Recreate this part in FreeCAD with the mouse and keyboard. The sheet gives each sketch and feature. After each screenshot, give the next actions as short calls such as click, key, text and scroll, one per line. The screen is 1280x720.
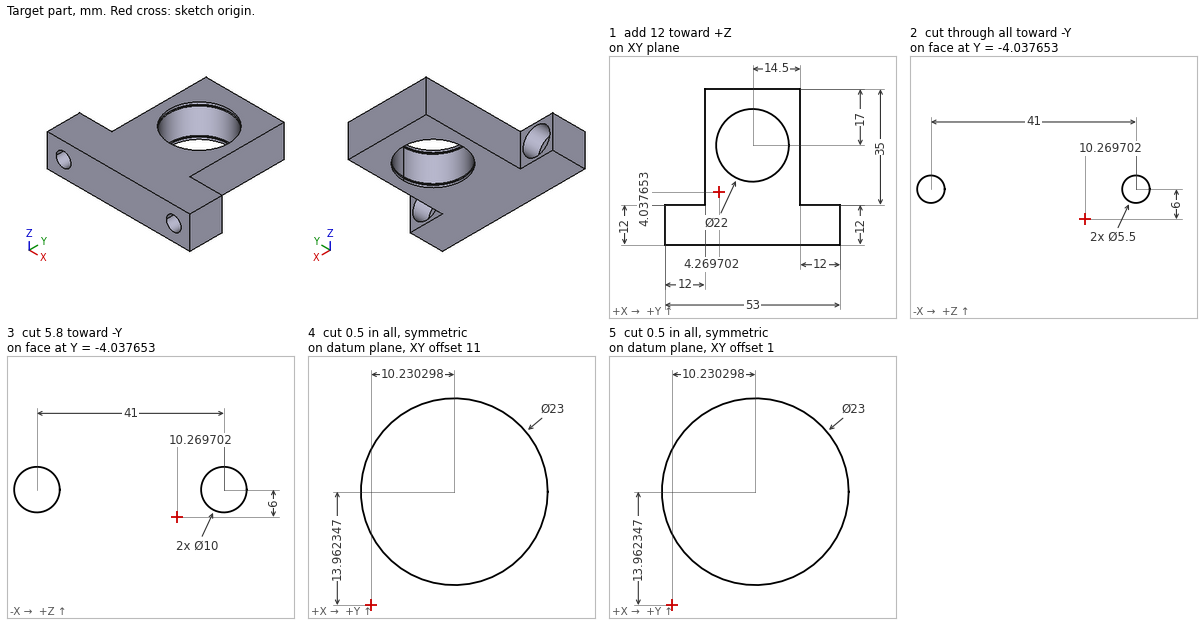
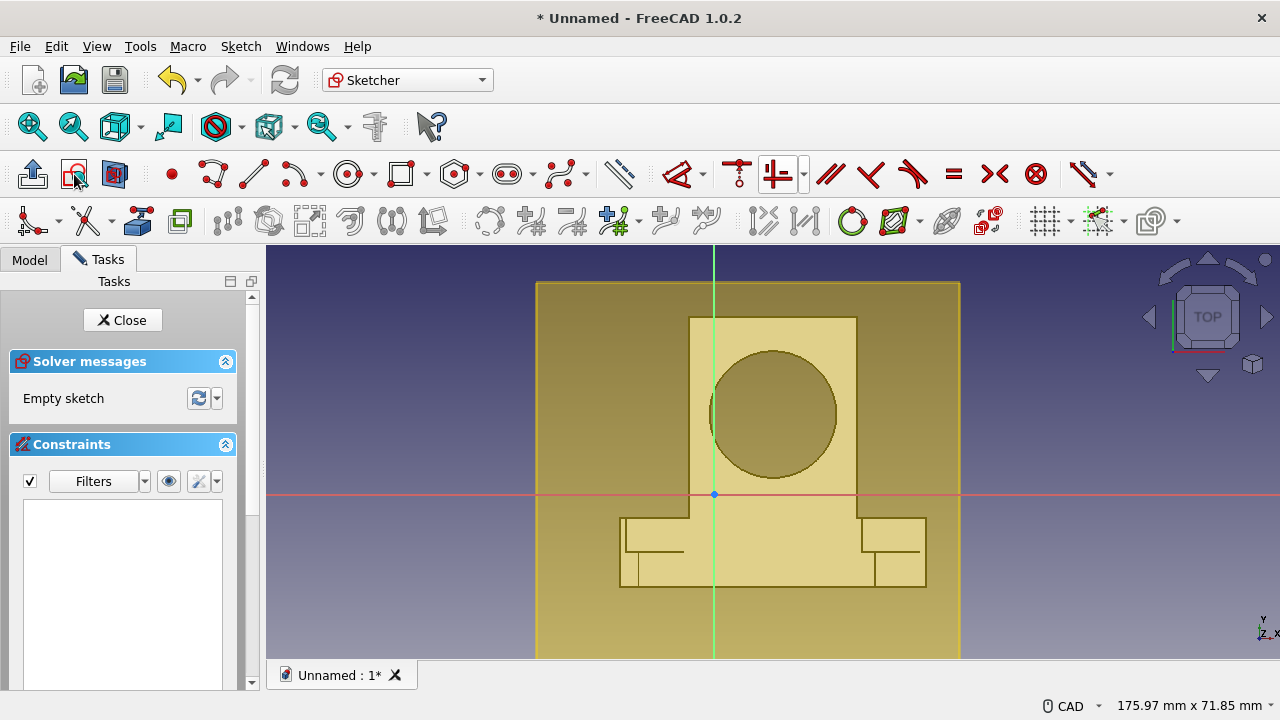
scroll(856, 385, up, 3)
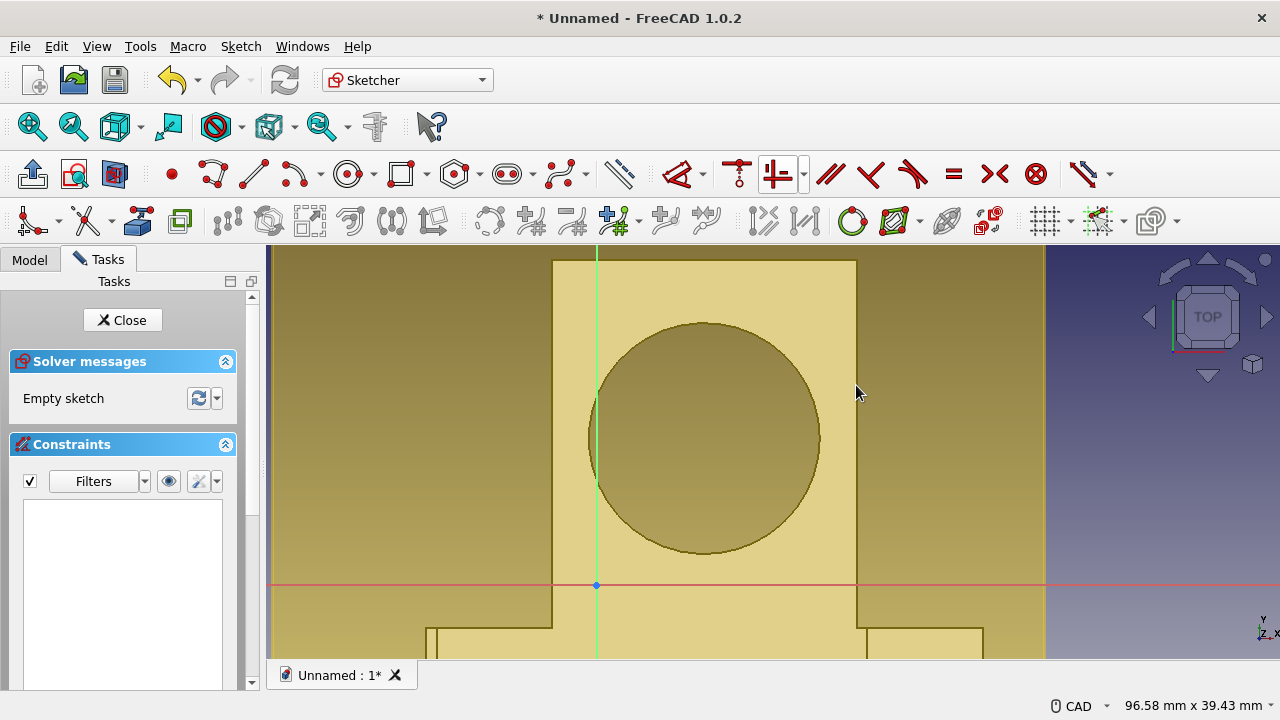
click(348, 174)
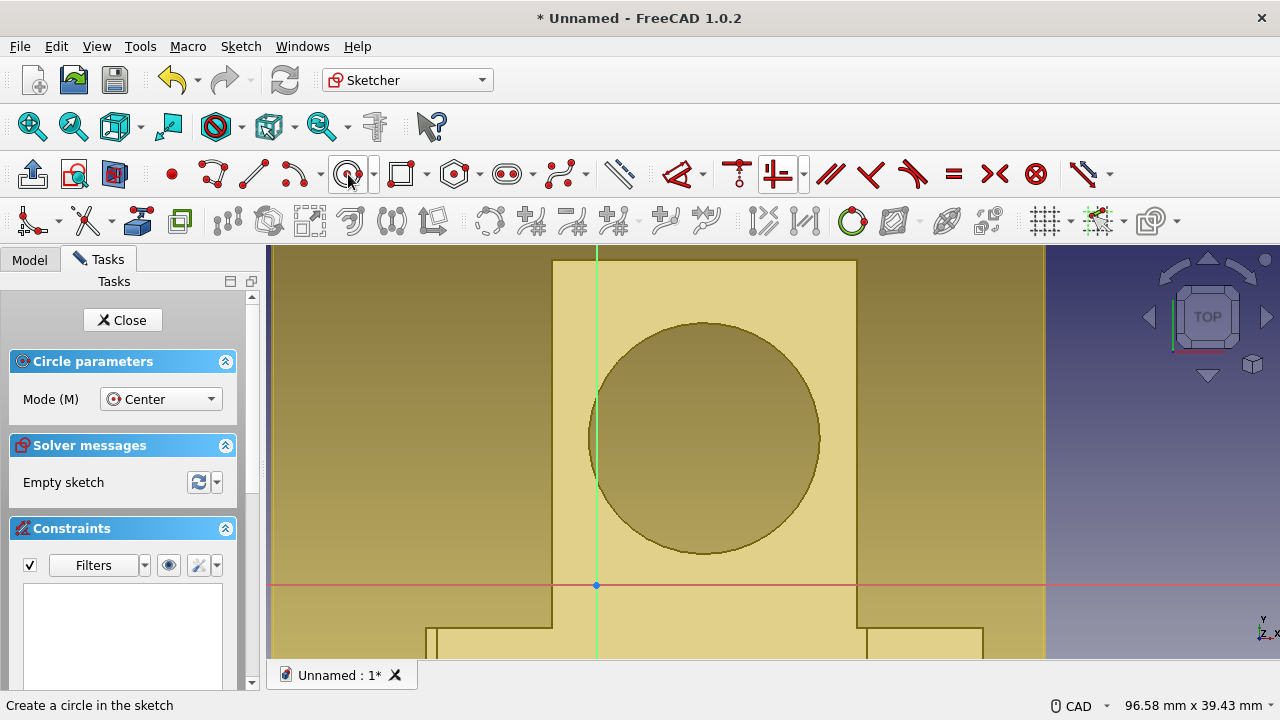
click(704, 439)
click(790, 353)
key(Escape)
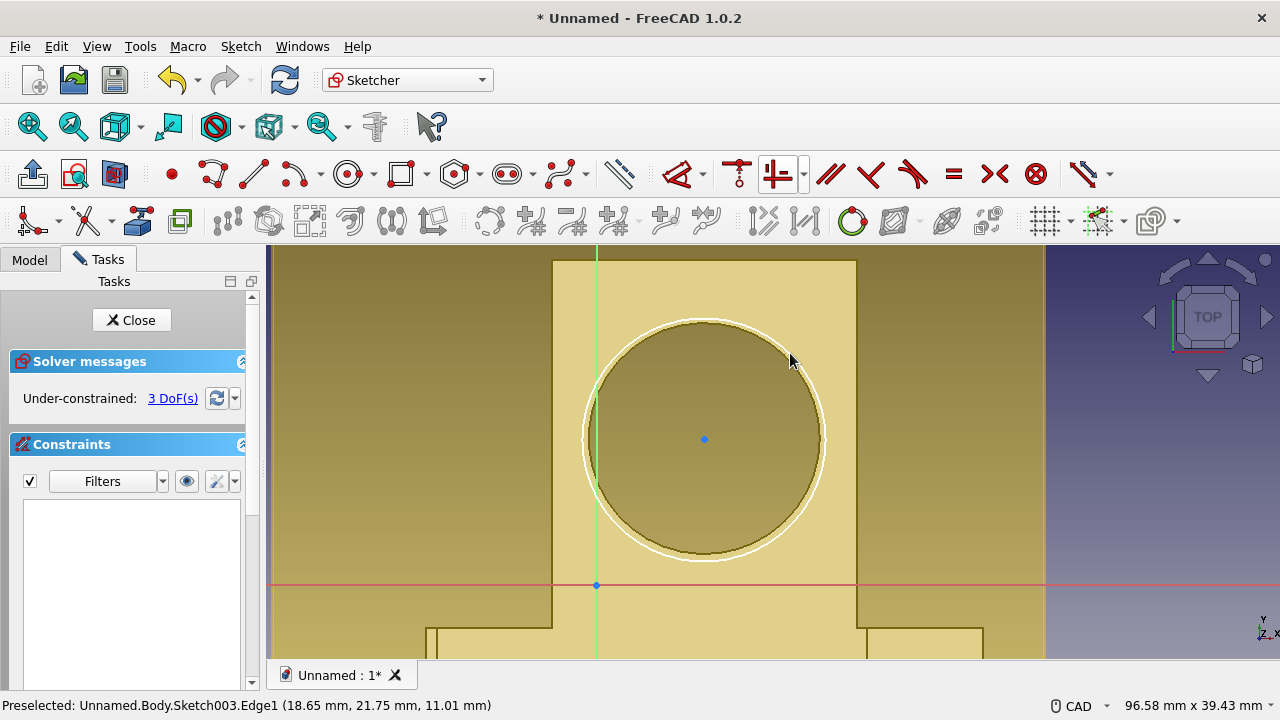
key(d)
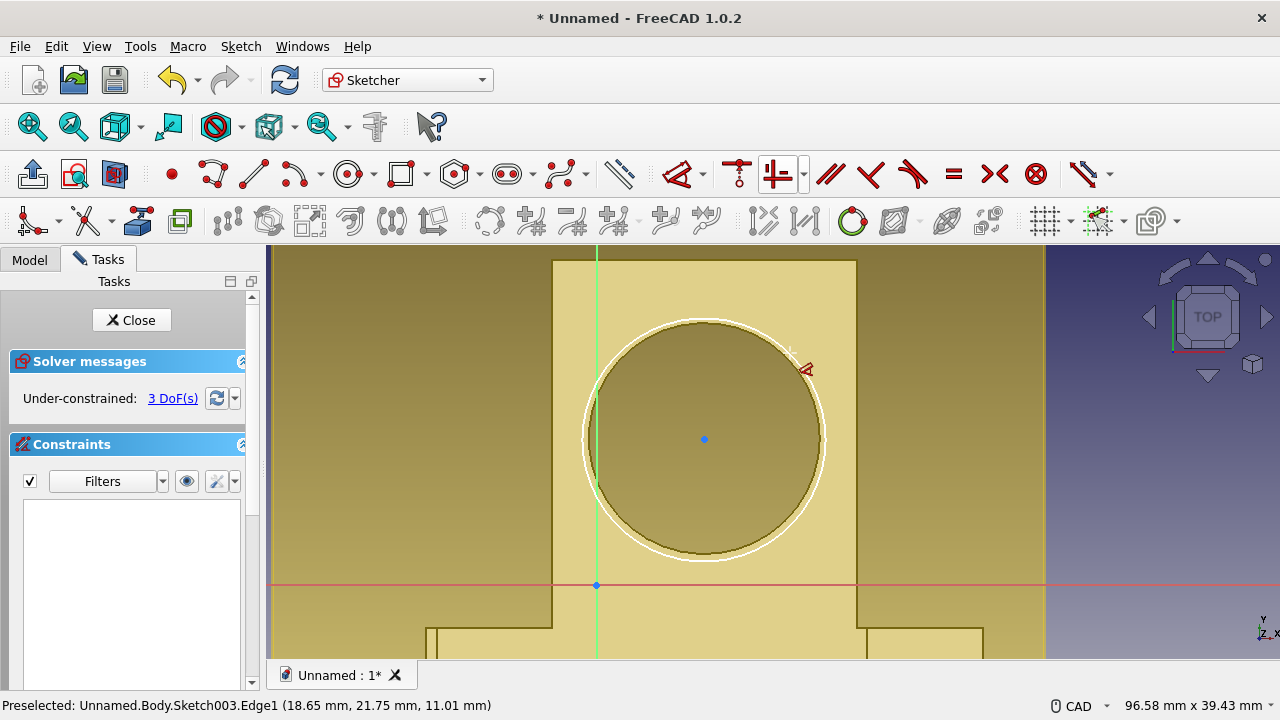
click(790, 354)
click(813, 331)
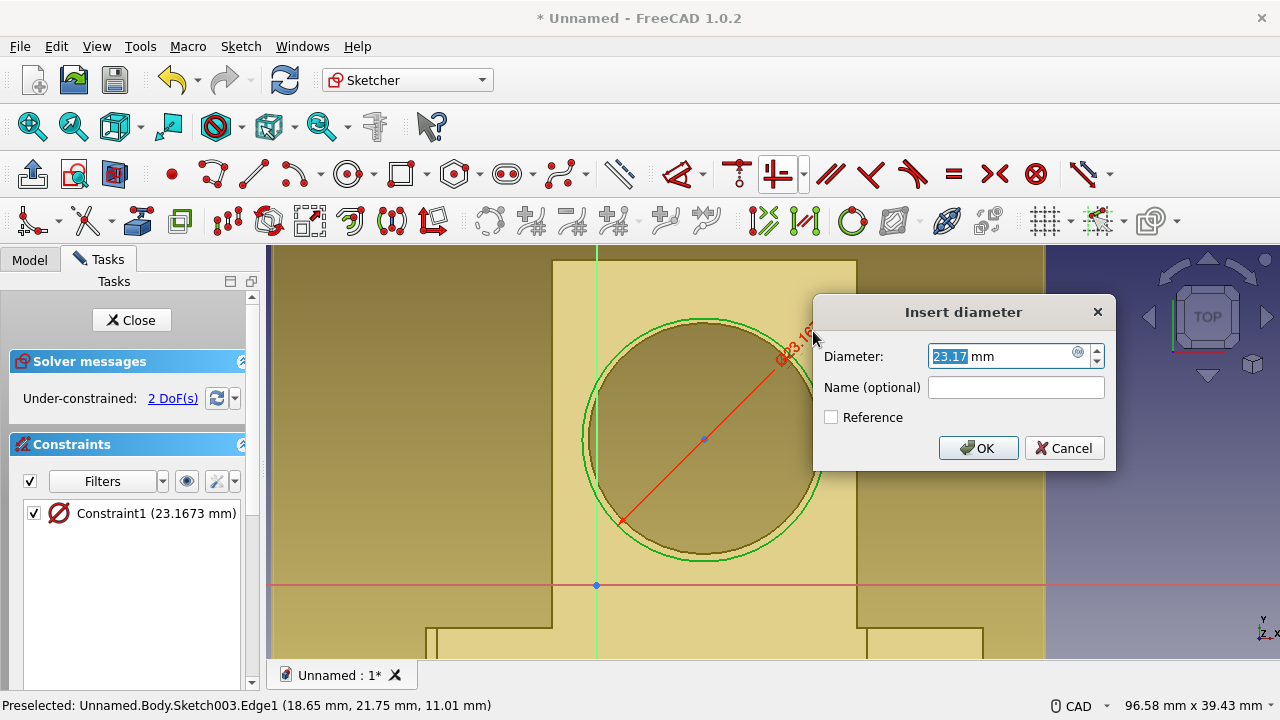
text(23)
key(Return)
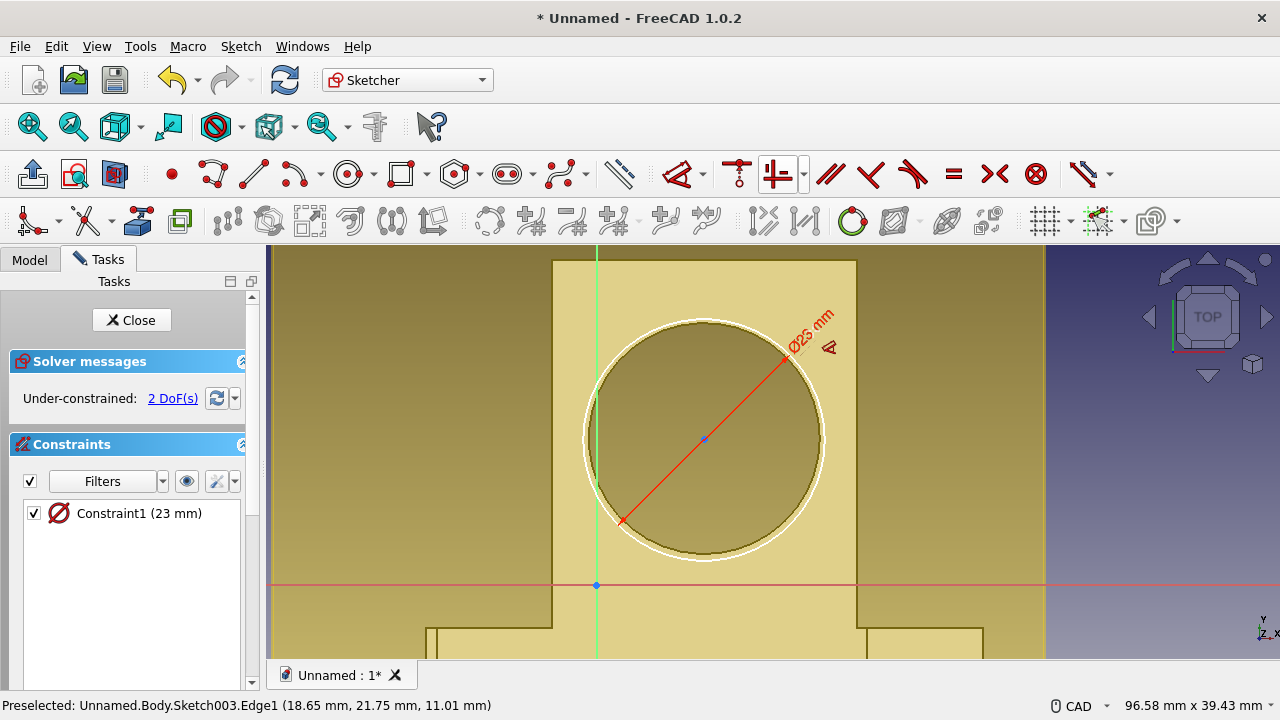
click(704, 440)
click(650, 619)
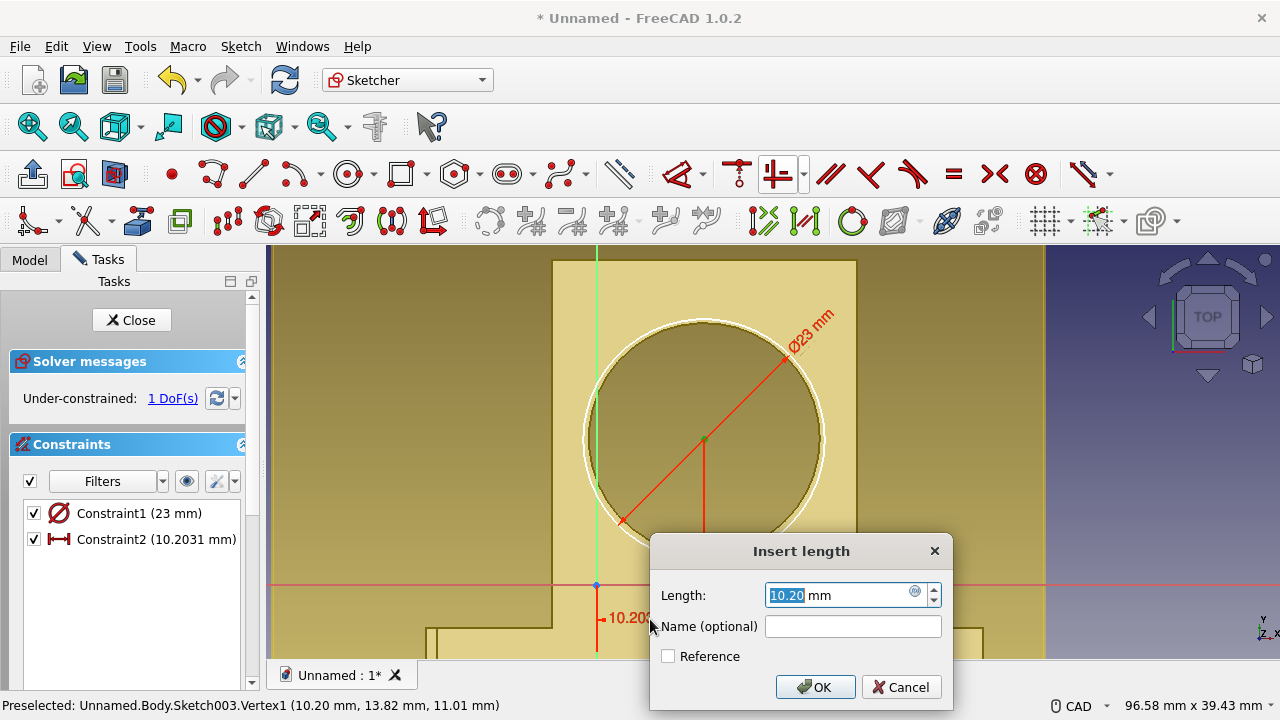
text(10.230298)
key(Return)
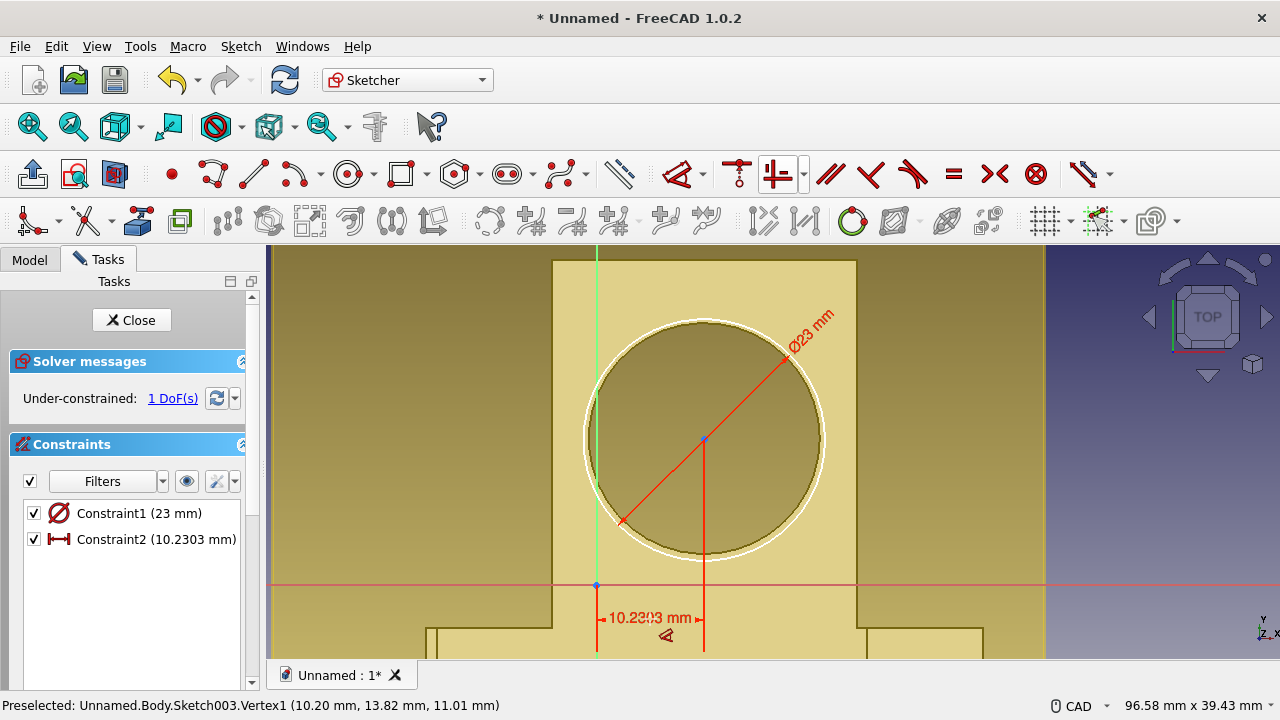
click(704, 440)
click(563, 513)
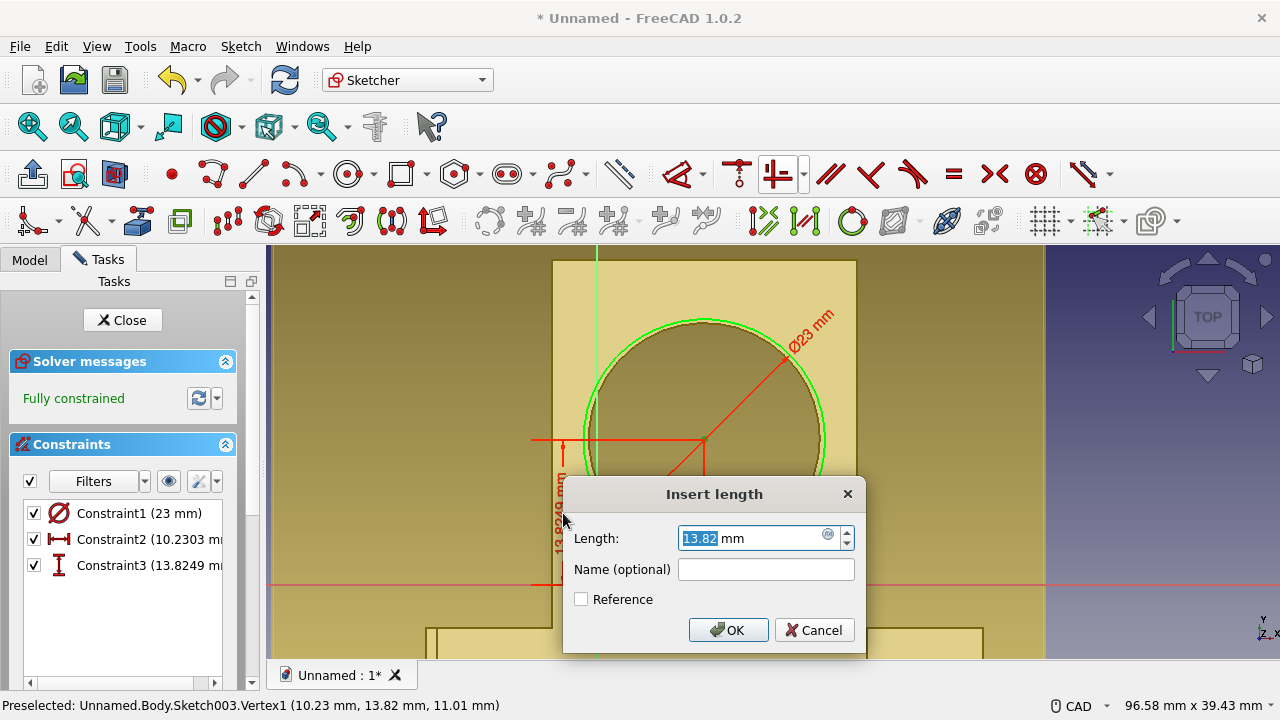
text(13.962347)
key(Return)
key(Escape)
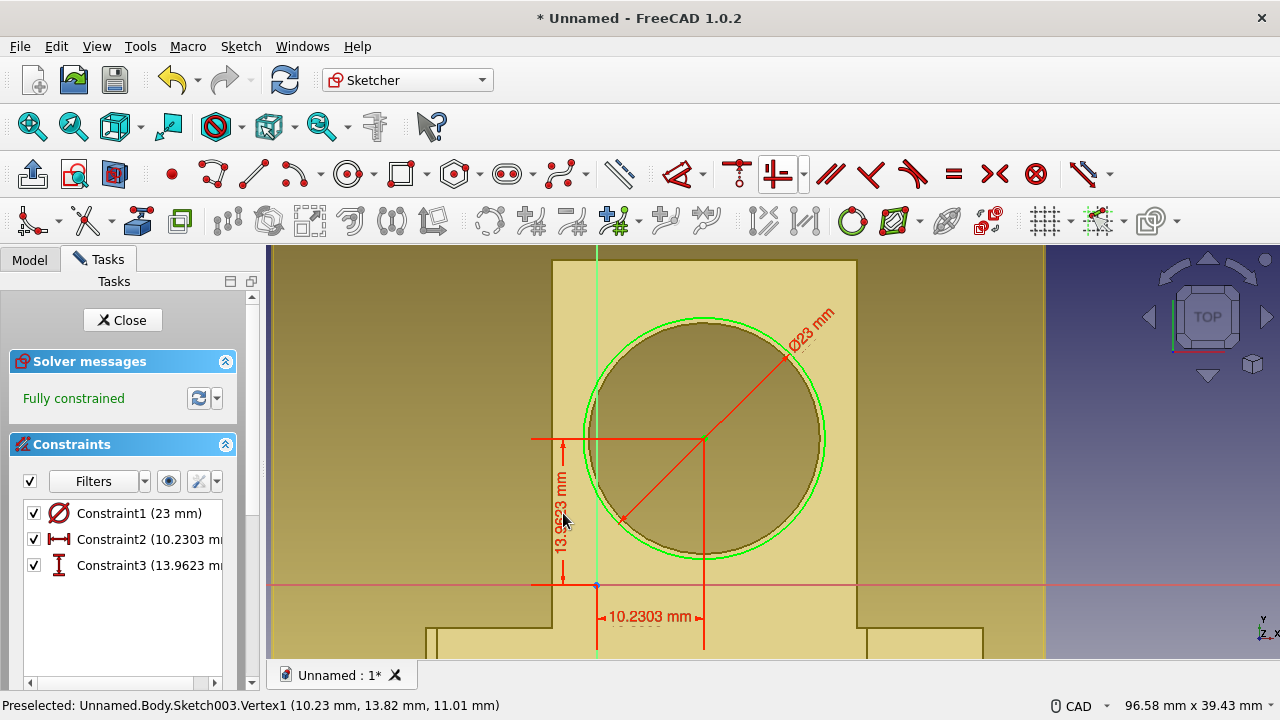
click(123, 320)